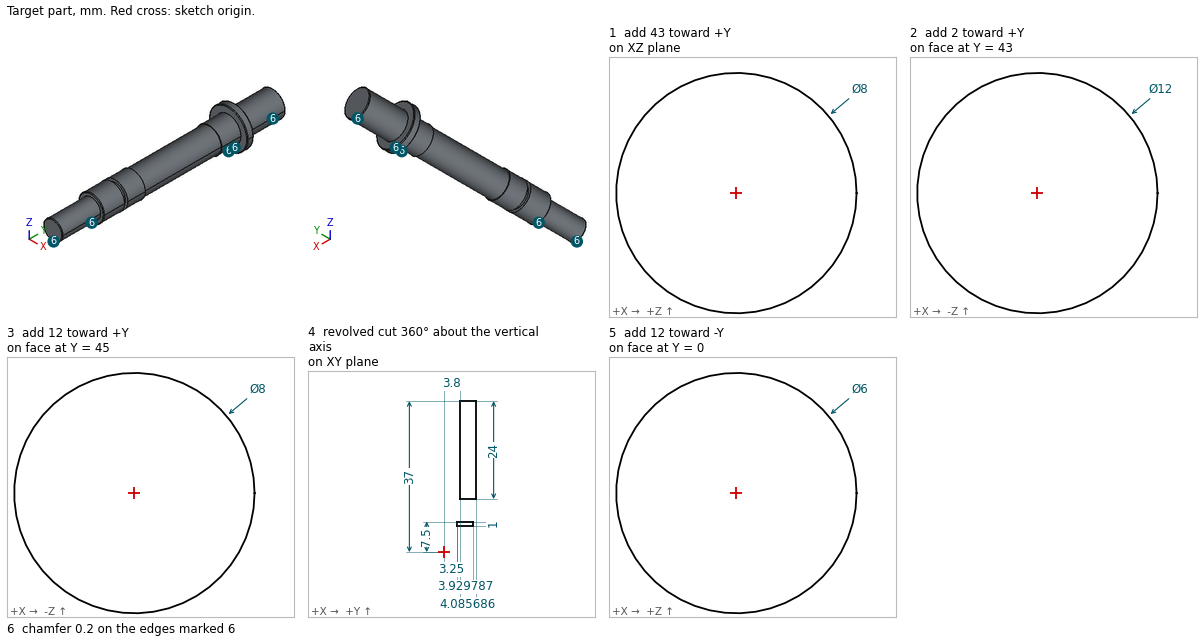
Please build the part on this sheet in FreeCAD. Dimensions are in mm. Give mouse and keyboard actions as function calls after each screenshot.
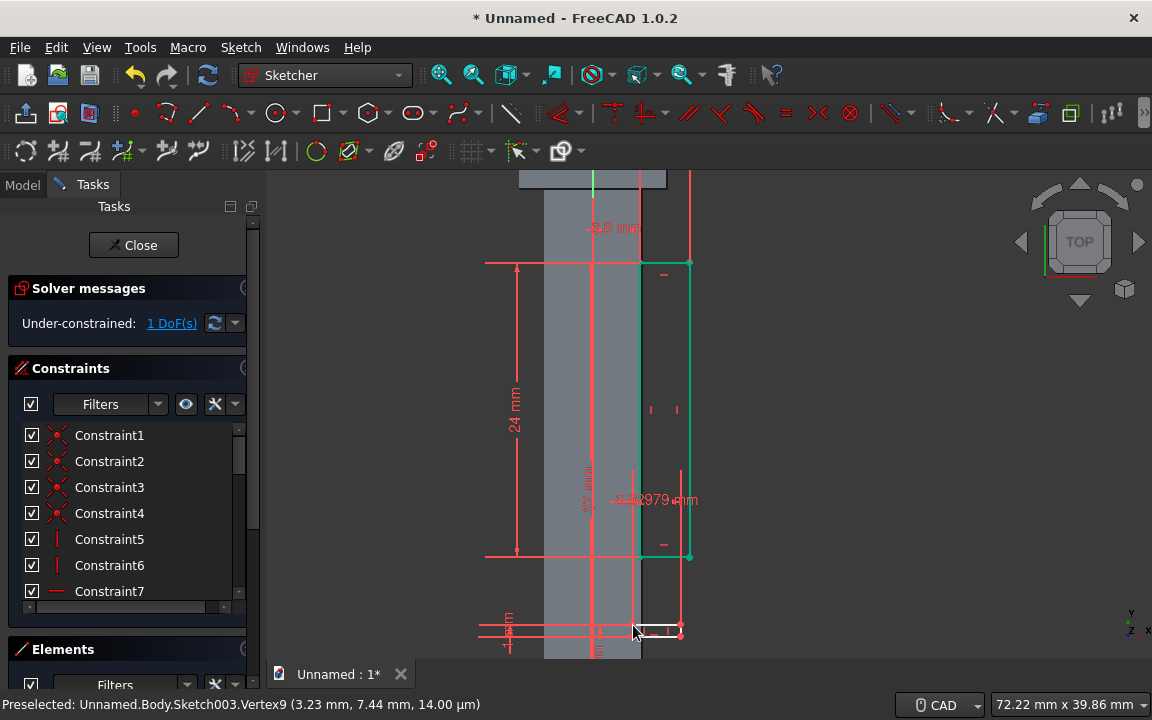
click(633, 625)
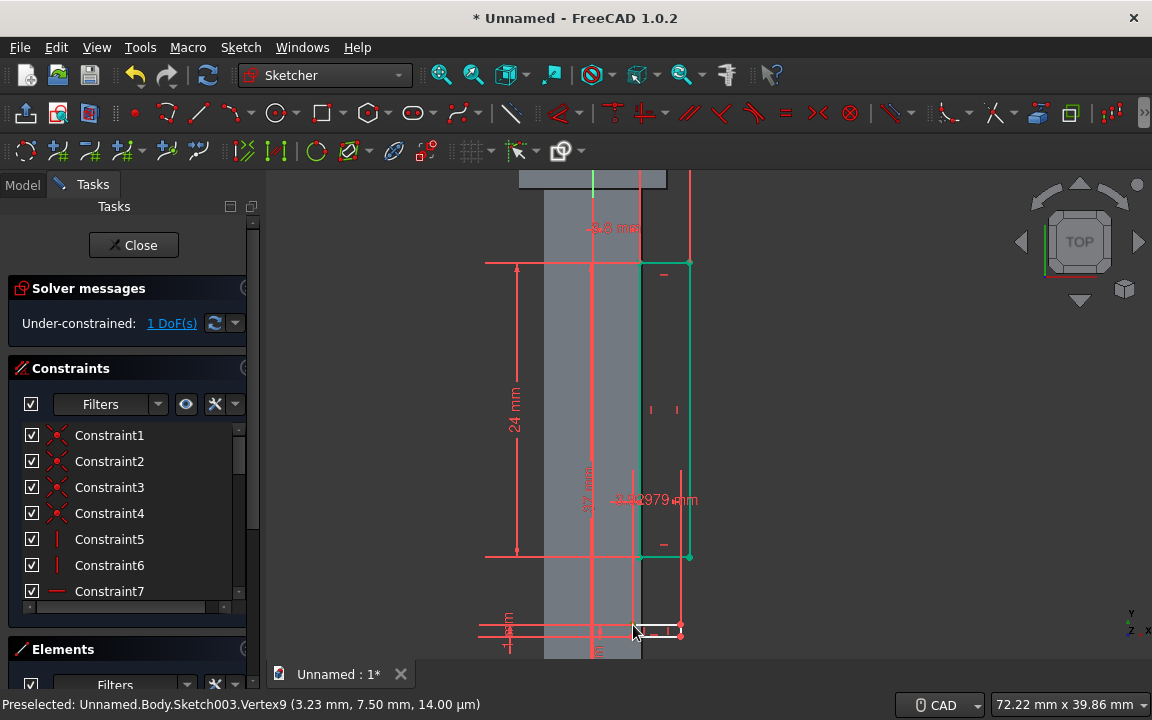
click(582, 114)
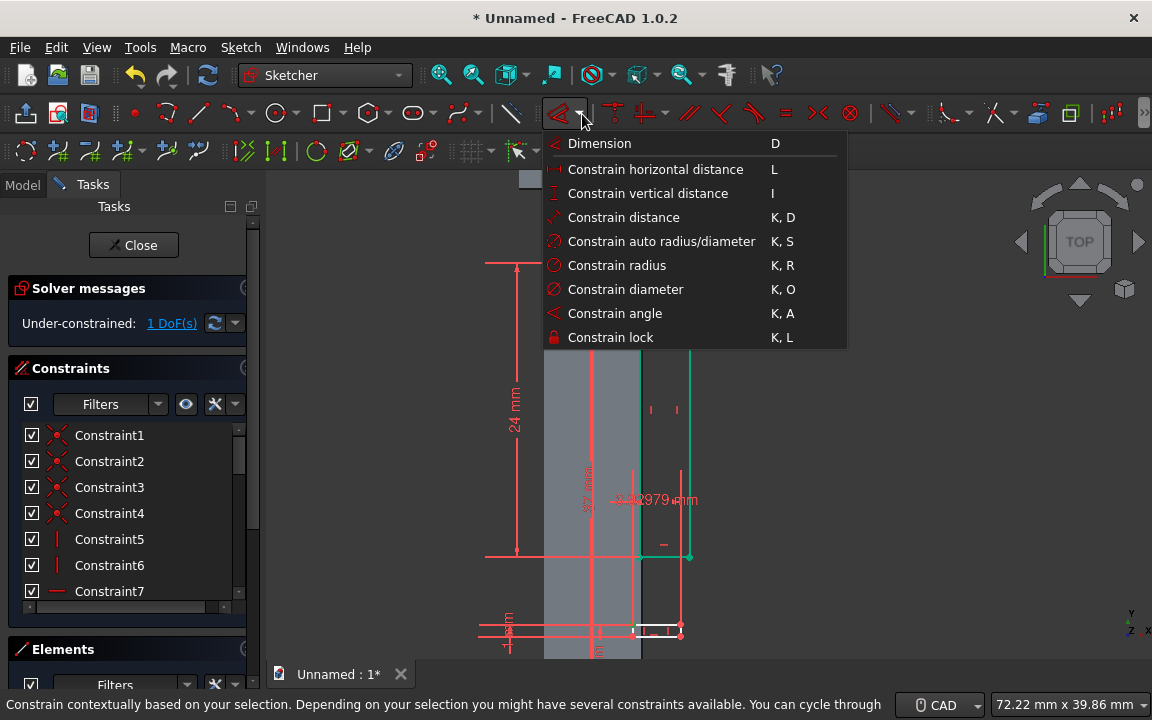
click(695, 169)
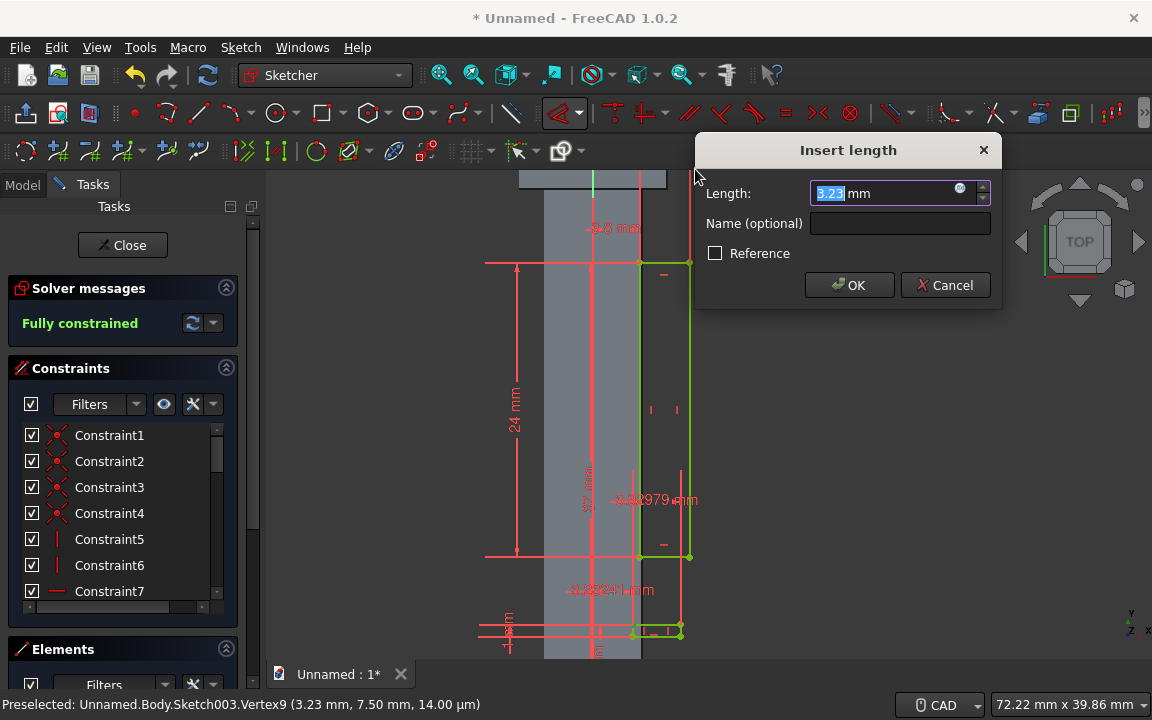
text(3.25)
key(Return)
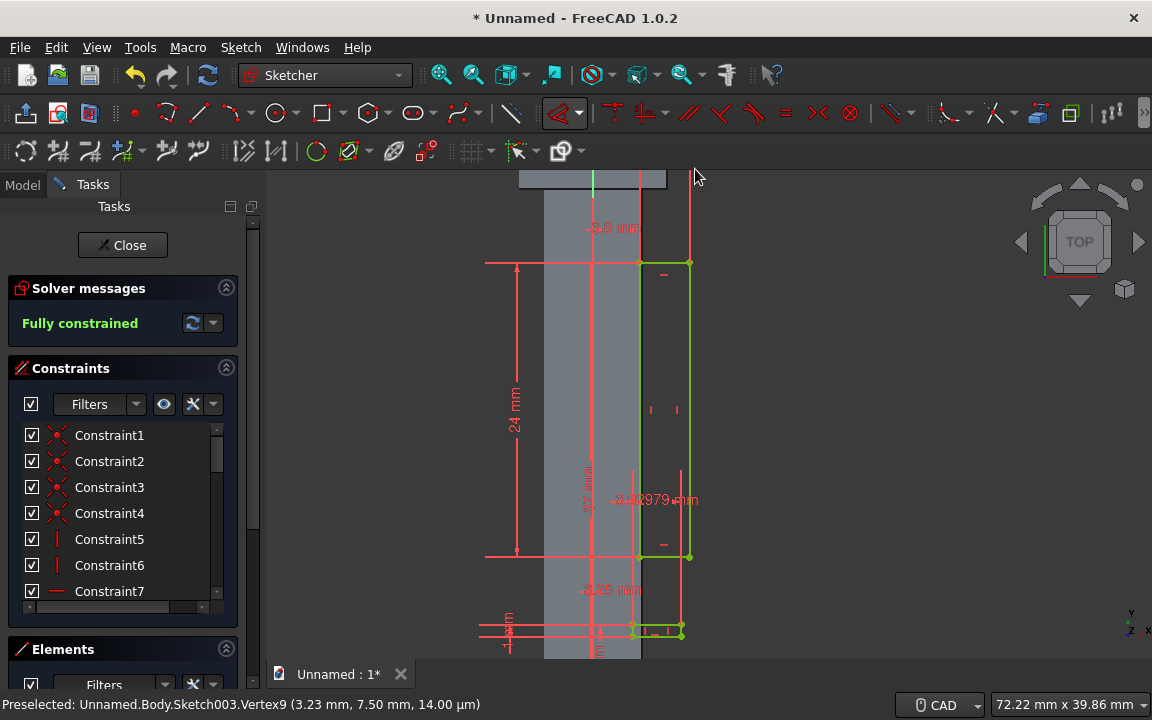
click(123, 245)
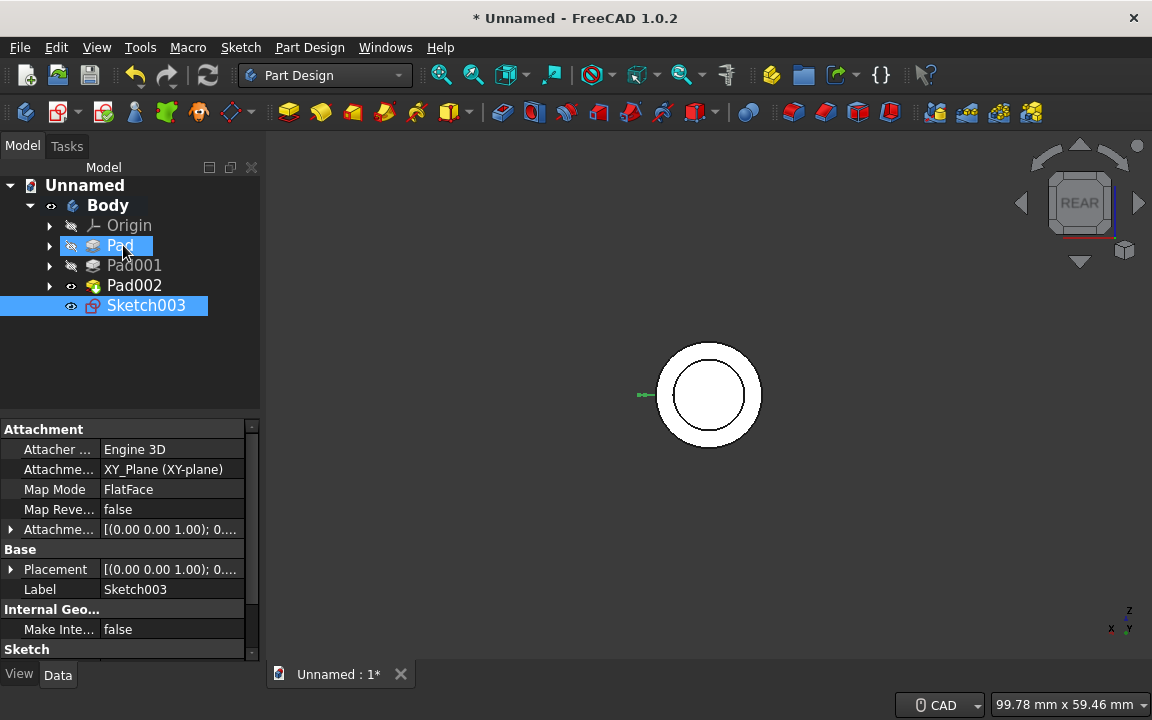
click(568, 112)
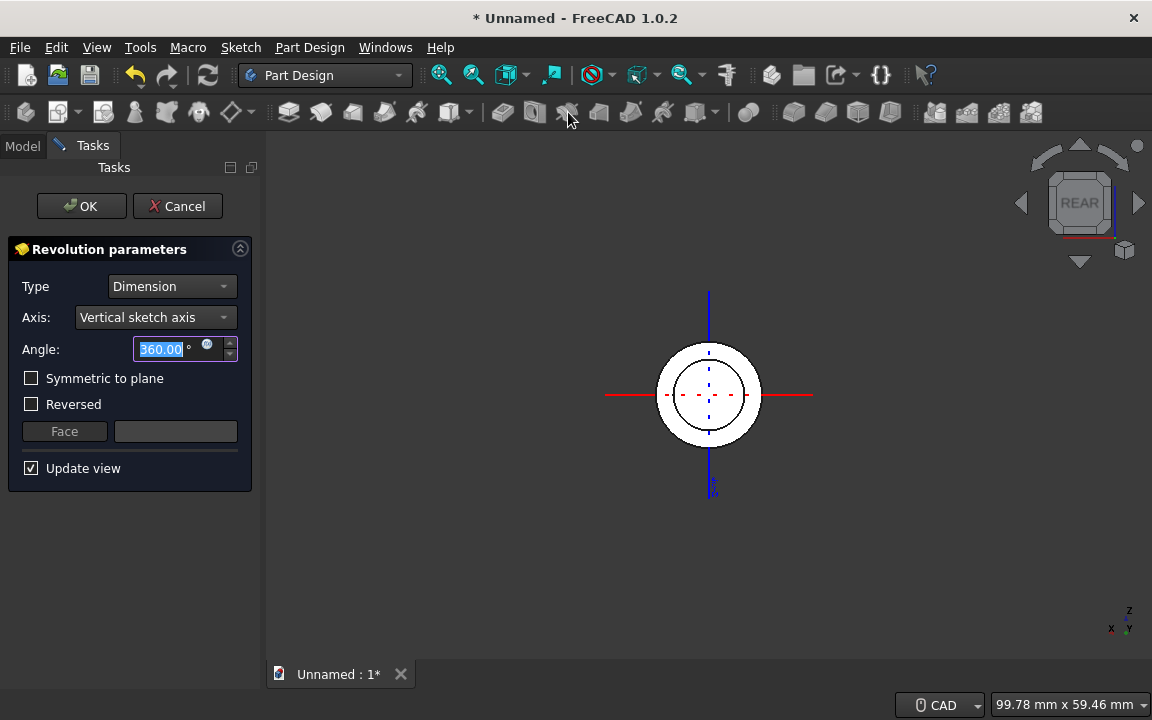
click(82, 206)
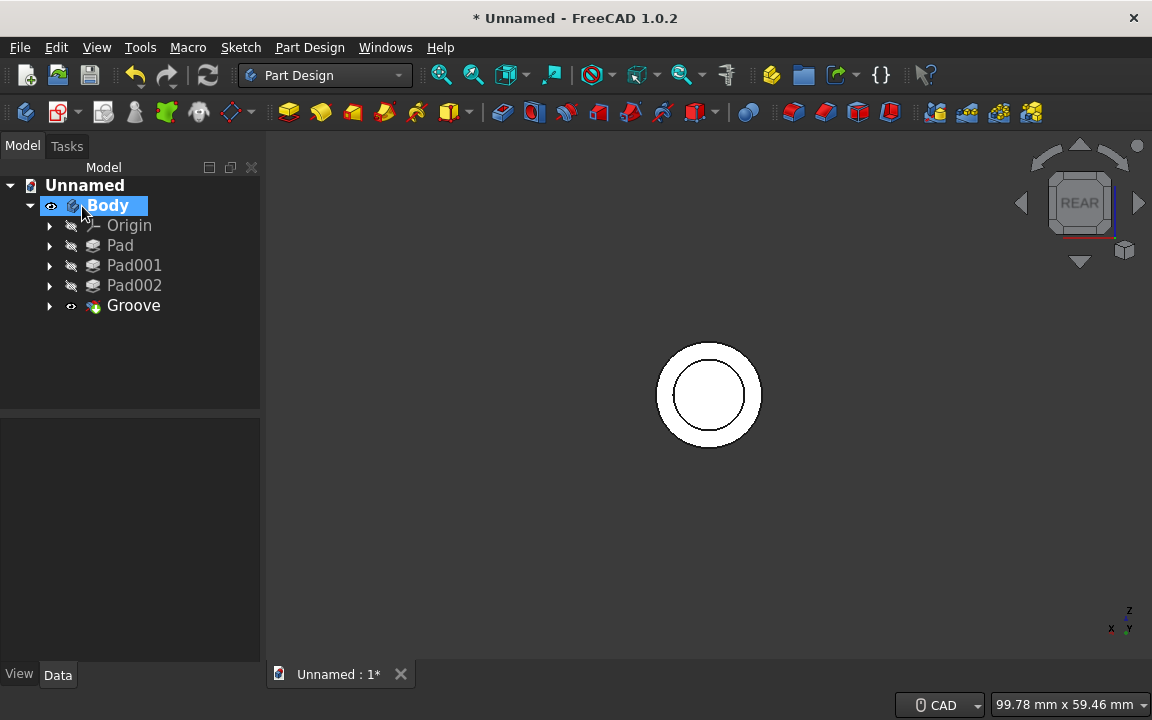
click(442, 76)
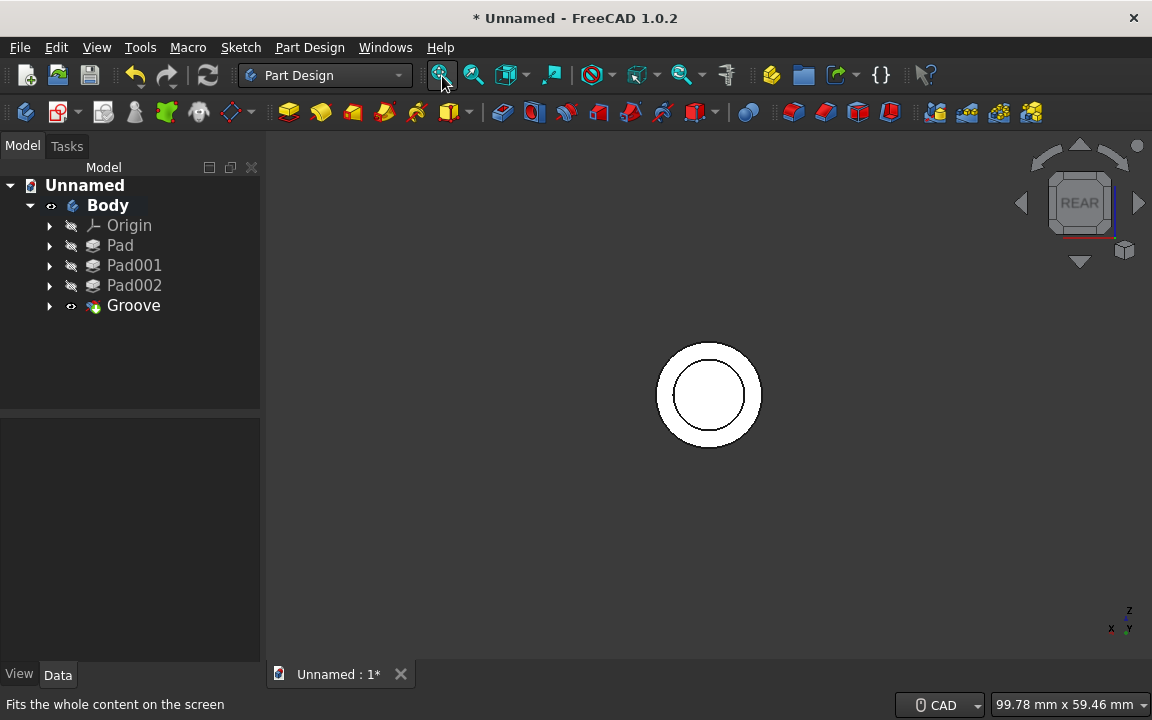
key(0)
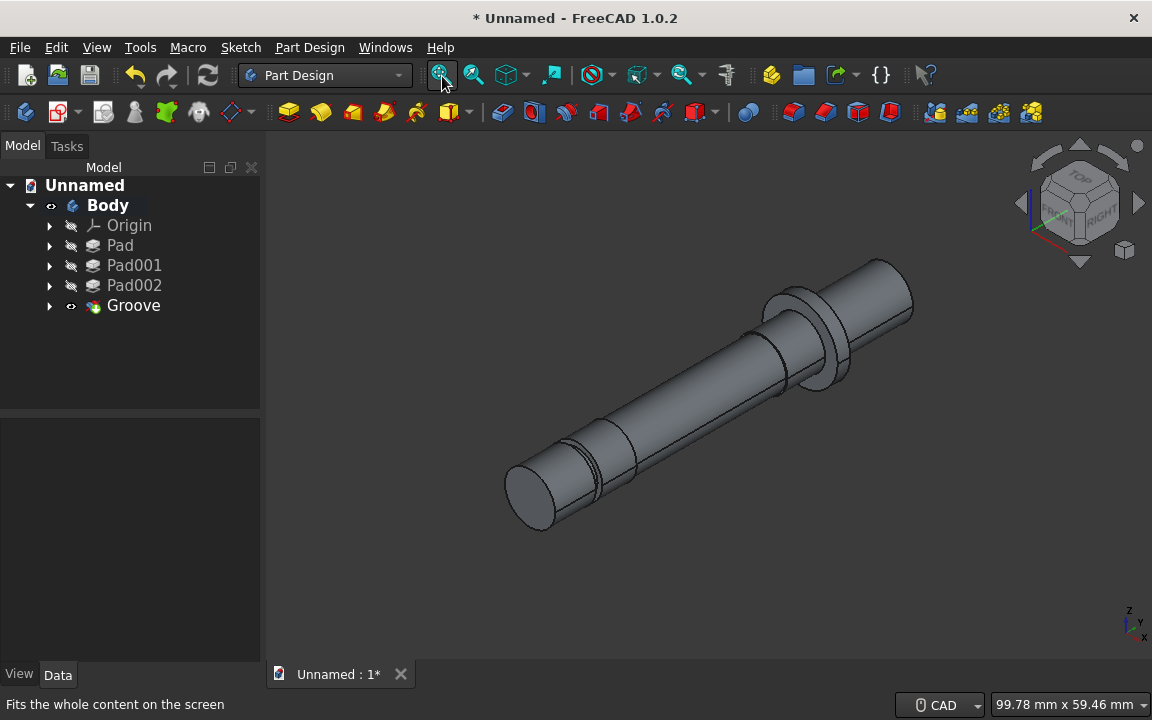
click(530, 497)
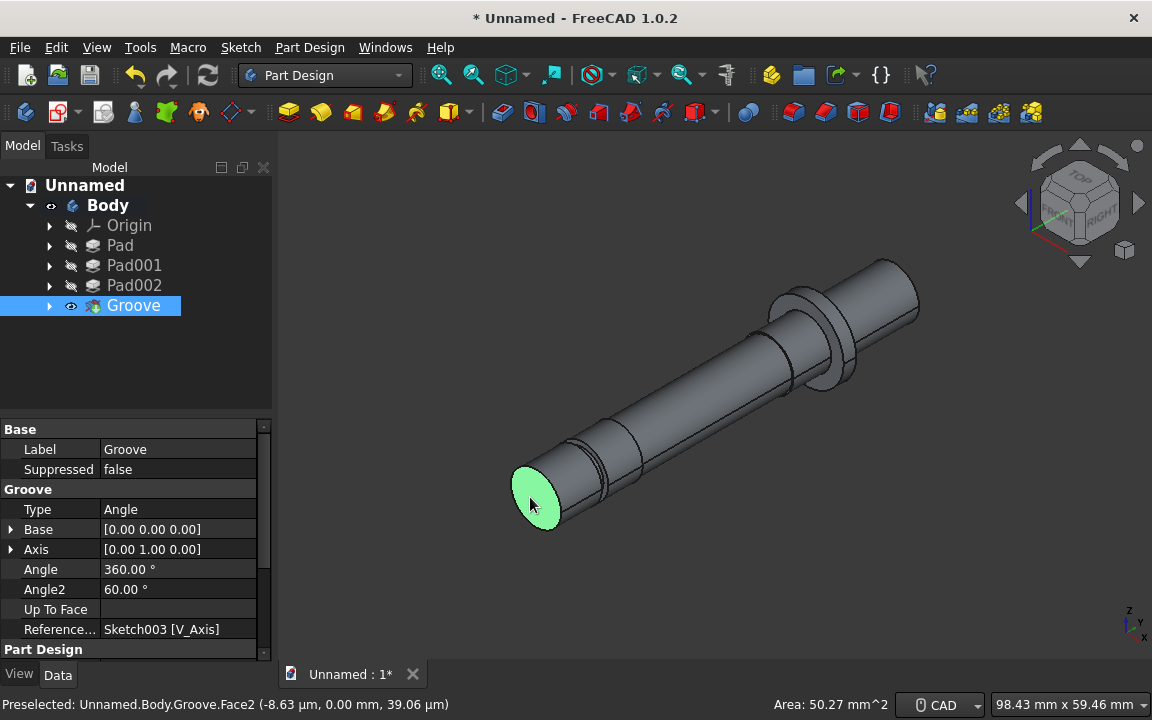
click(58, 112)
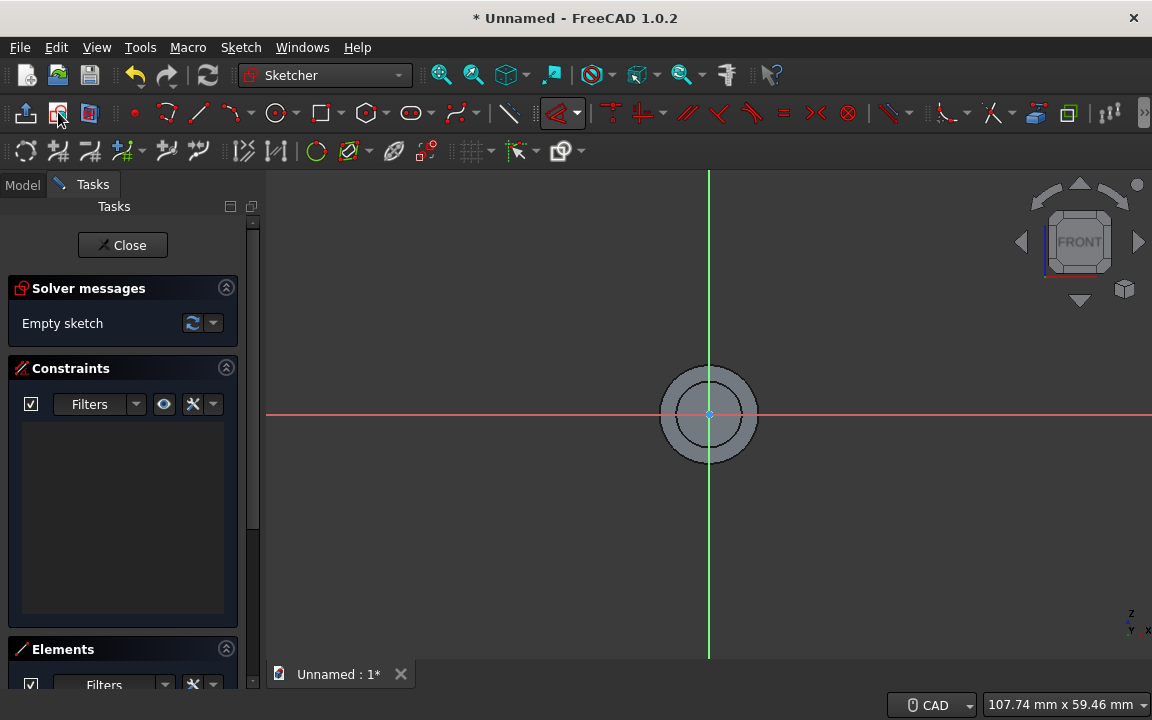
scroll(723, 415, up, 9)